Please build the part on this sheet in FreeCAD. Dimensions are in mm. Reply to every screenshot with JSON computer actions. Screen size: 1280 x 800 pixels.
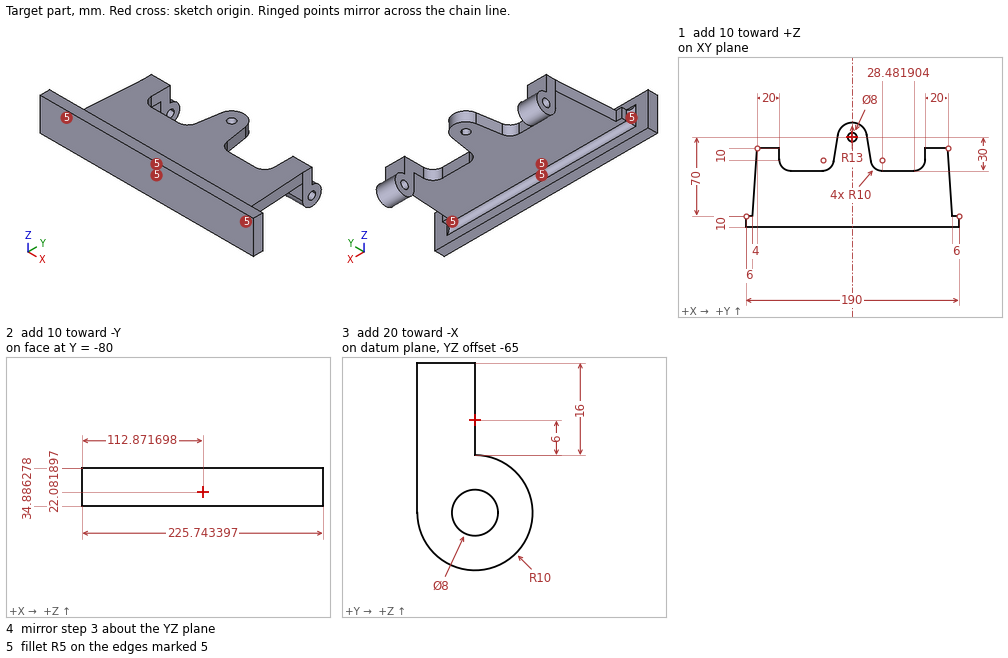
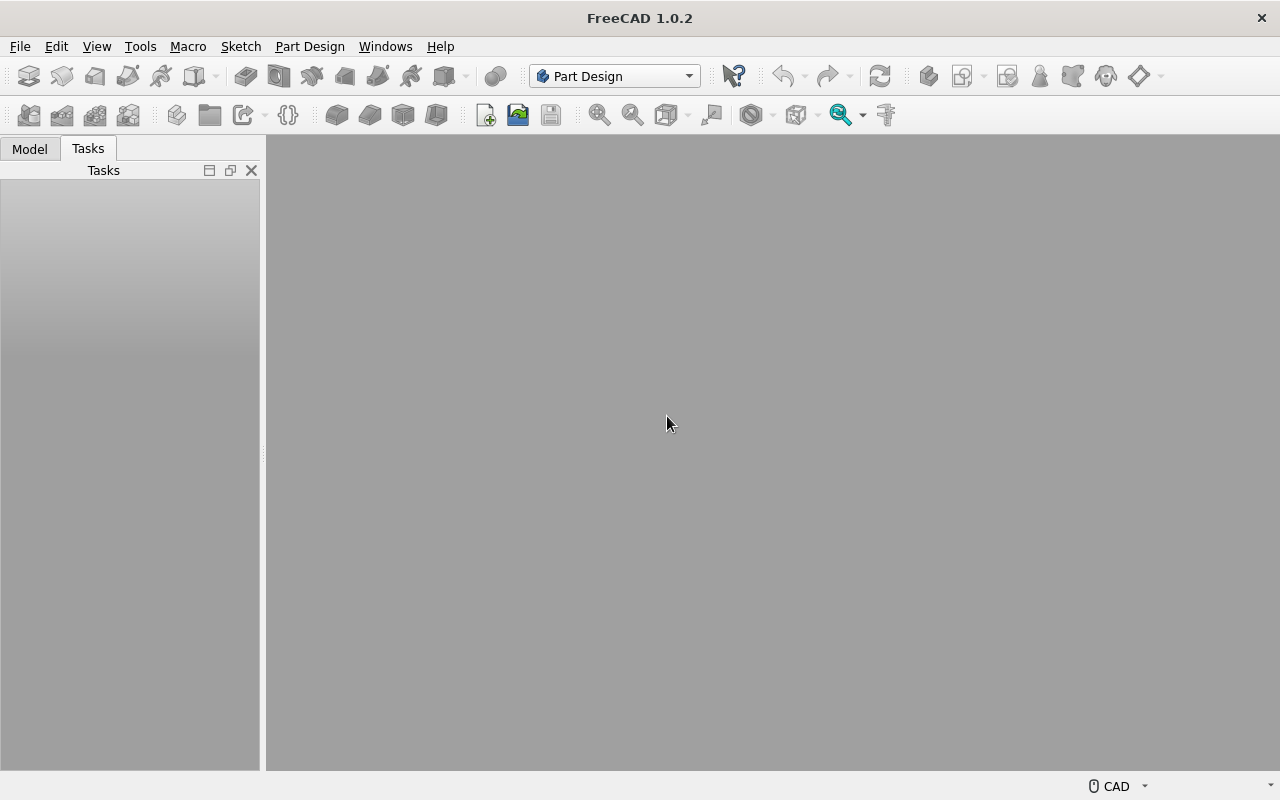
{"action": "left_click", "coordinate": [485, 116]}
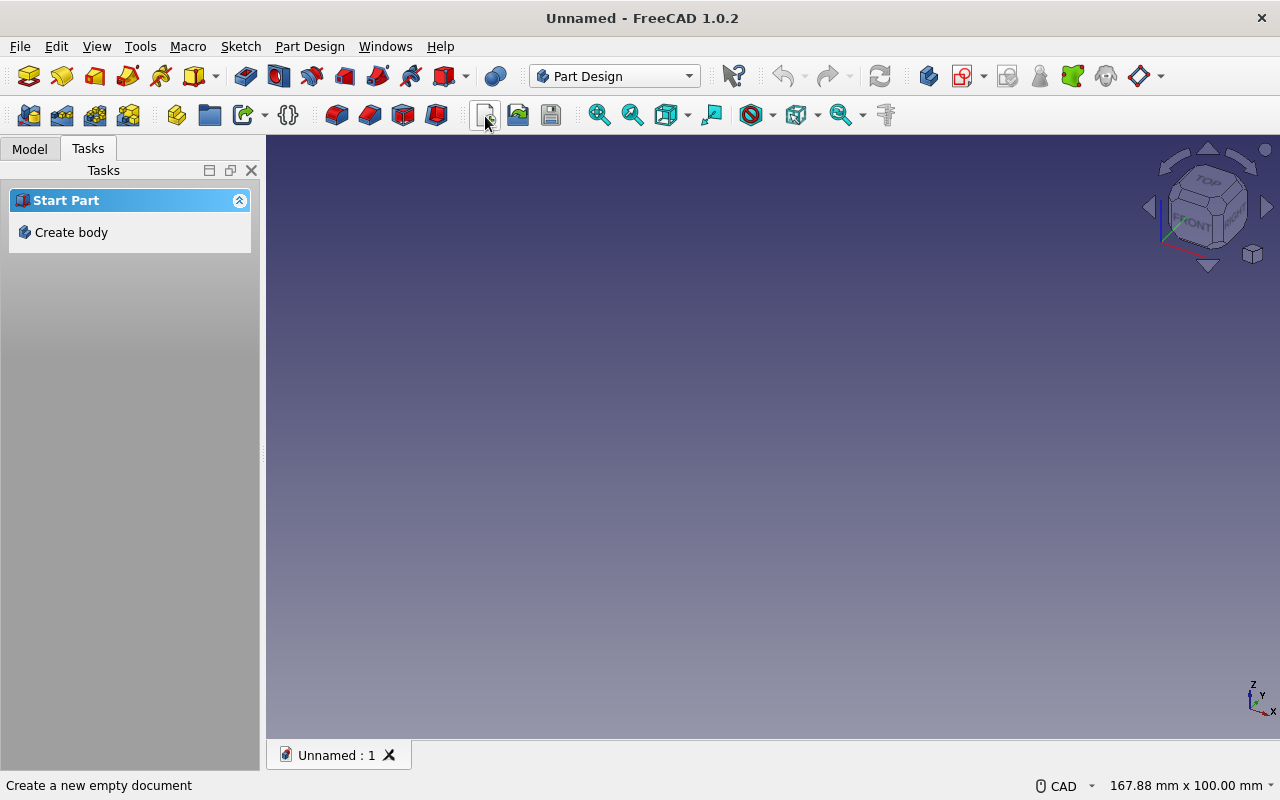
{"action": "left_click", "coordinate": [962, 76]}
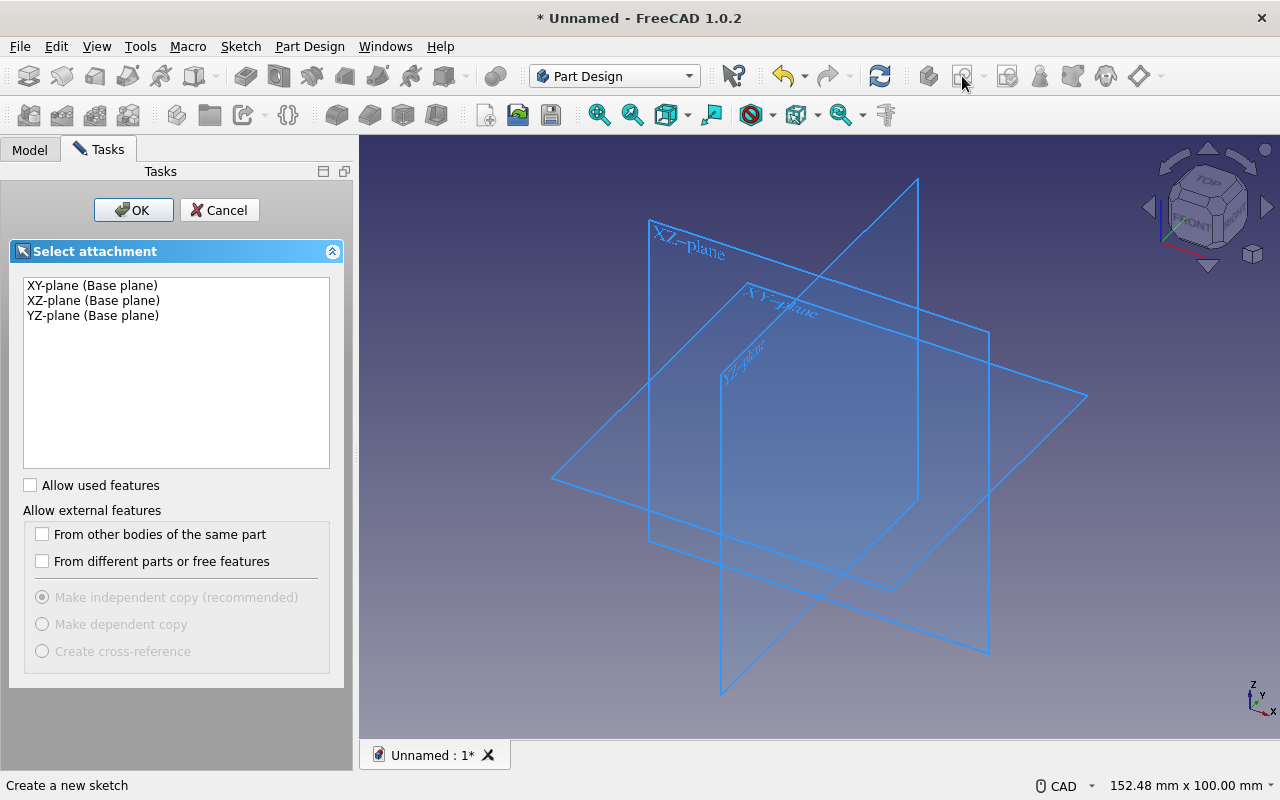
{"action": "left_click", "coordinate": [84, 286]}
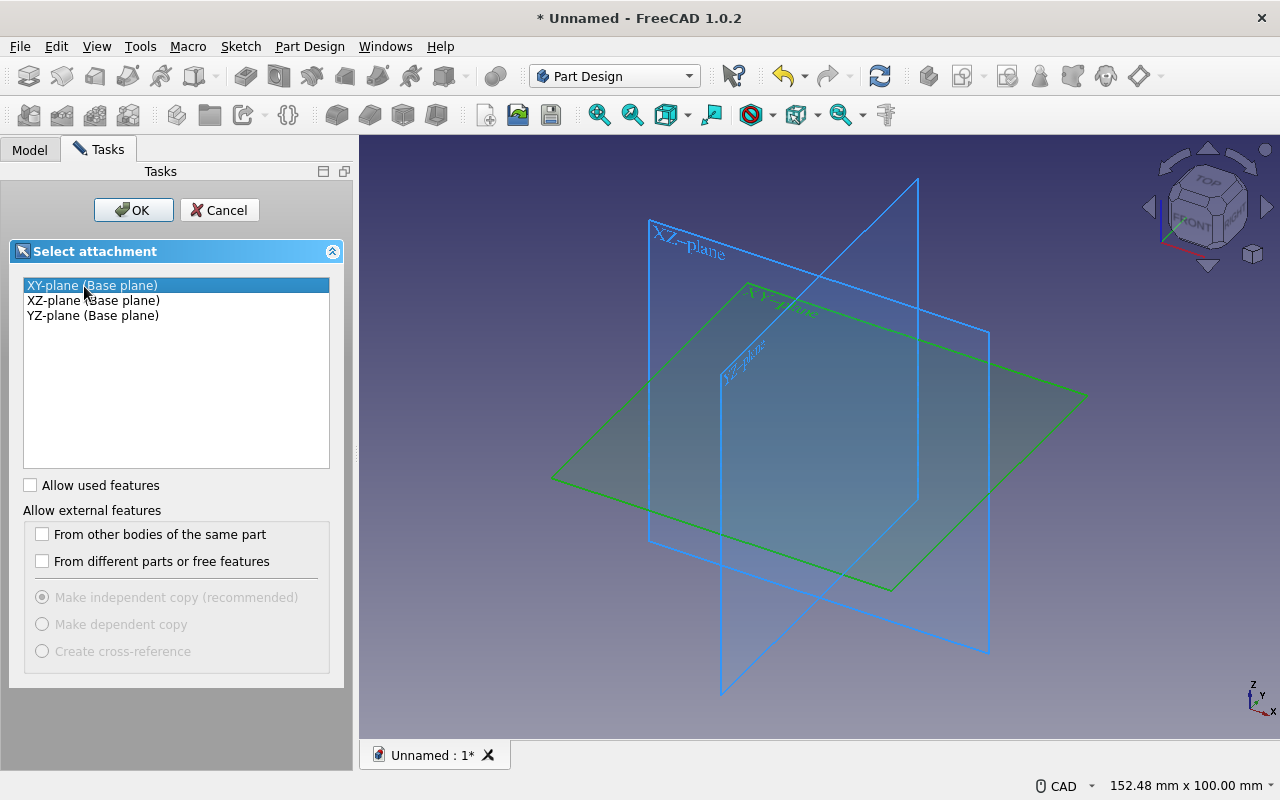
{"action": "left_click", "coordinate": [134, 210]}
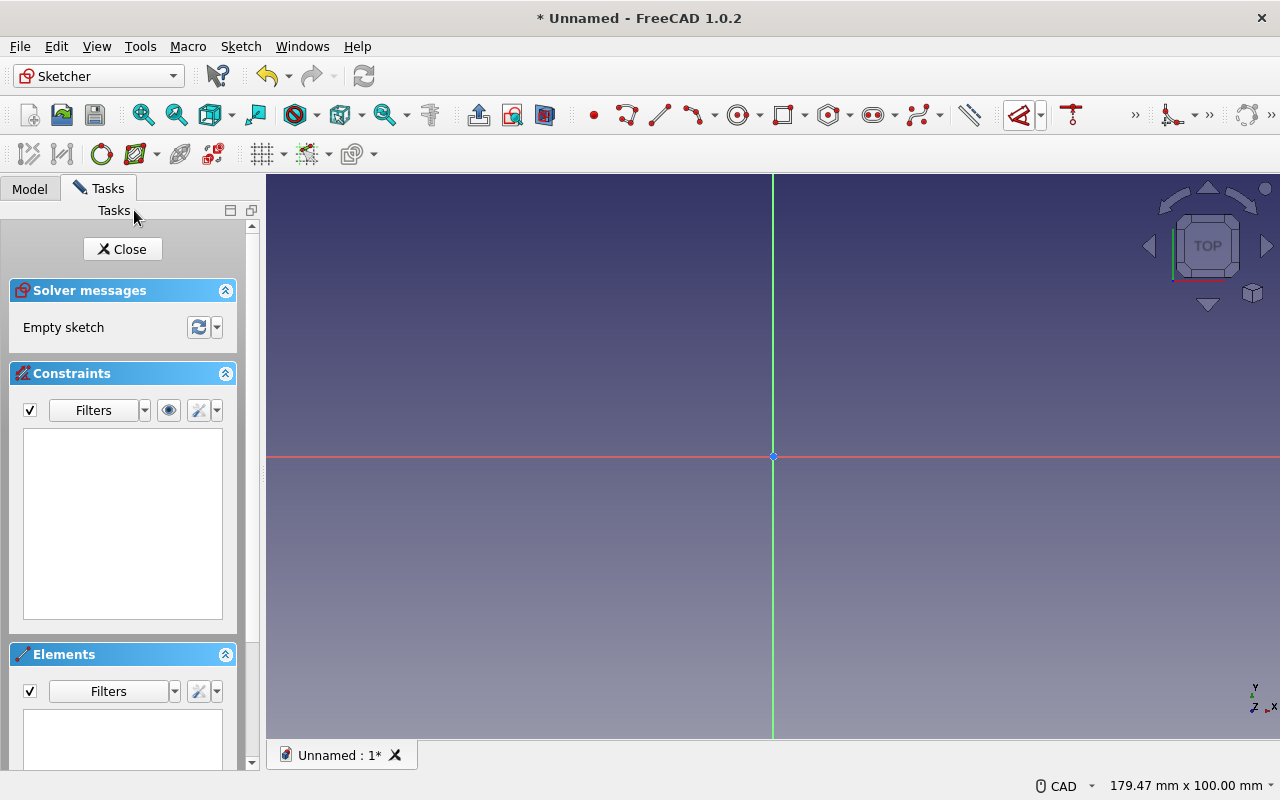
{"action": "scroll", "coordinate": [621, 226], "scroll_direction": "down", "scroll_amount": 3}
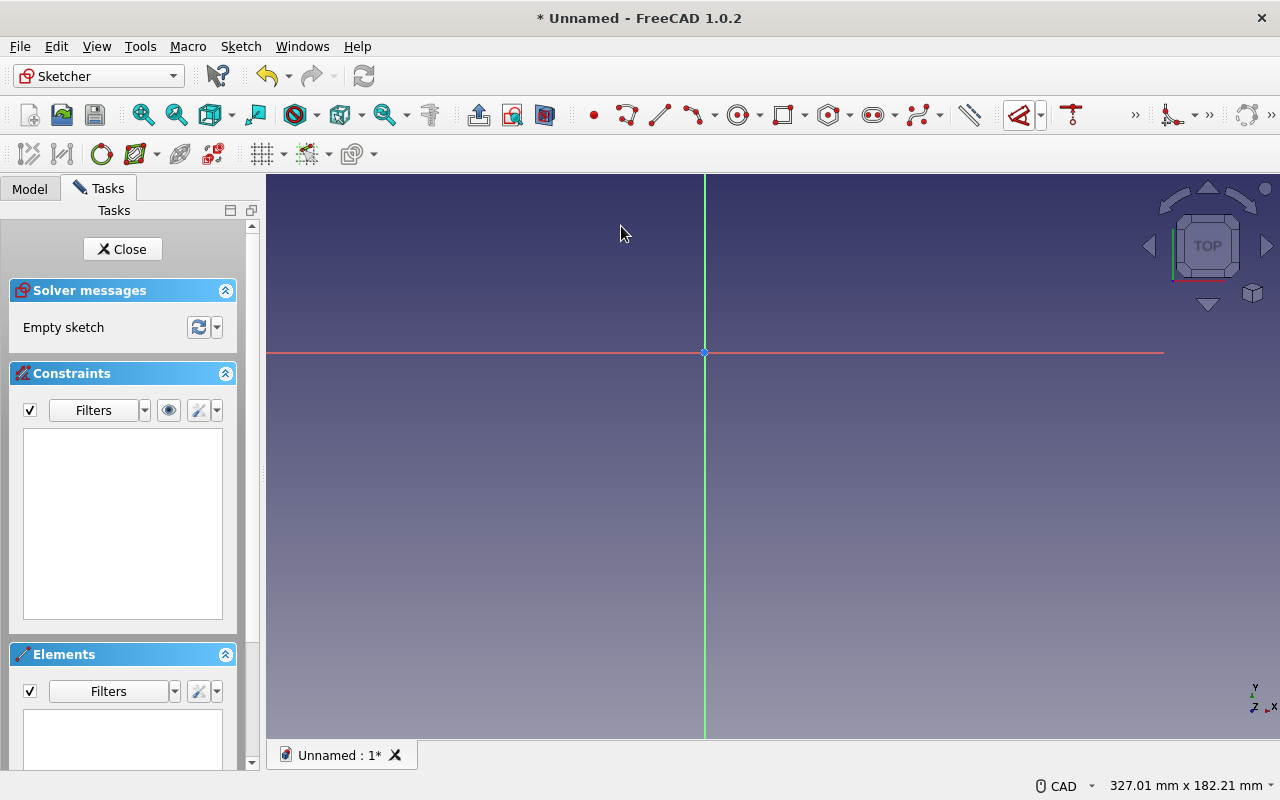
{"action": "left_click", "coordinate": [660, 116]}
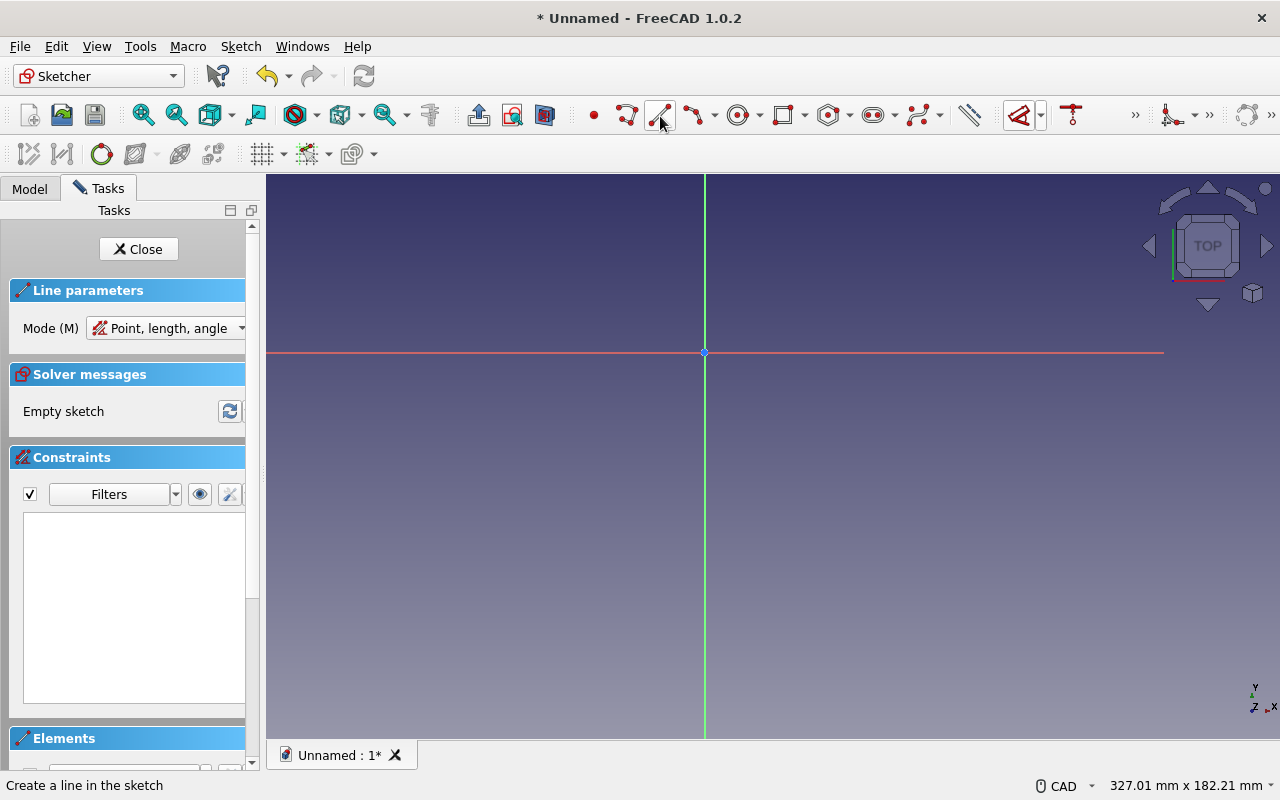
{"action": "left_click", "coordinate": [875, 446]}
{"action": "left_click", "coordinate": [787, 446]}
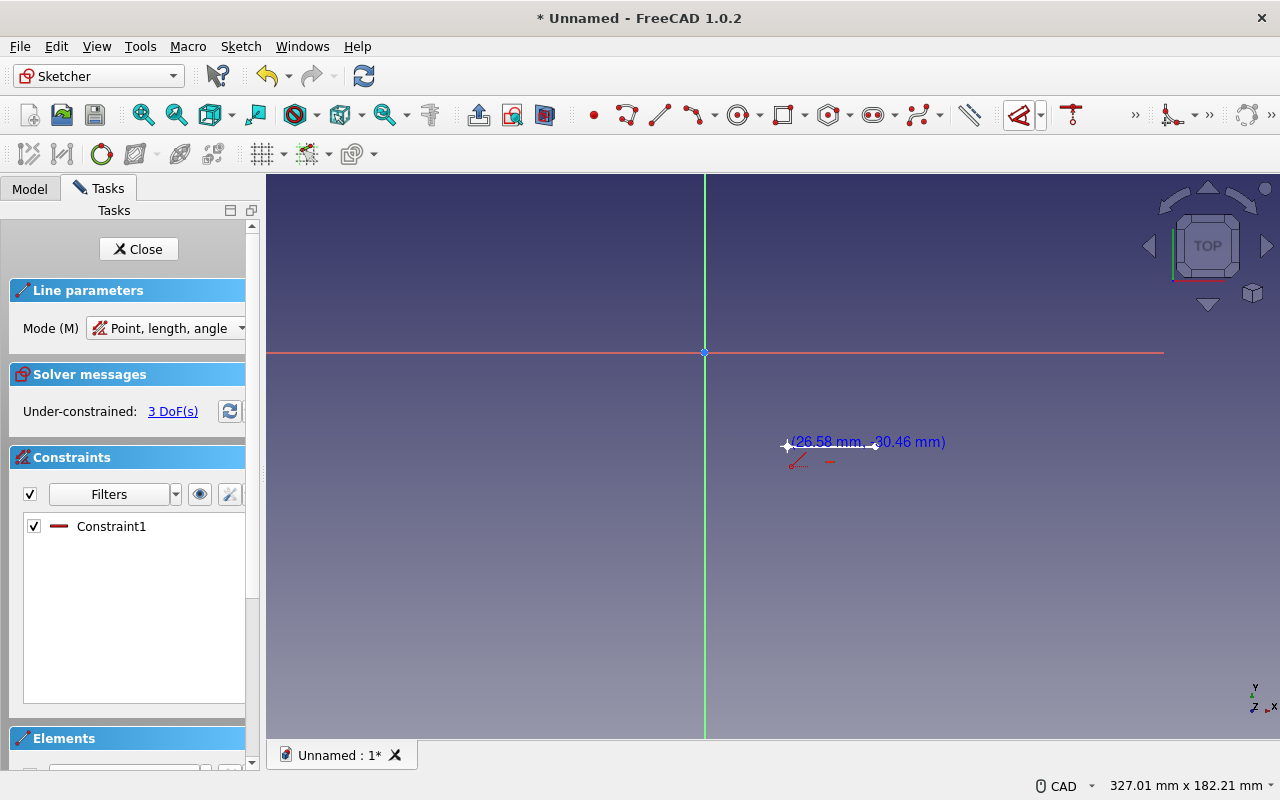
{"action": "left_click", "coordinate": [756, 419]}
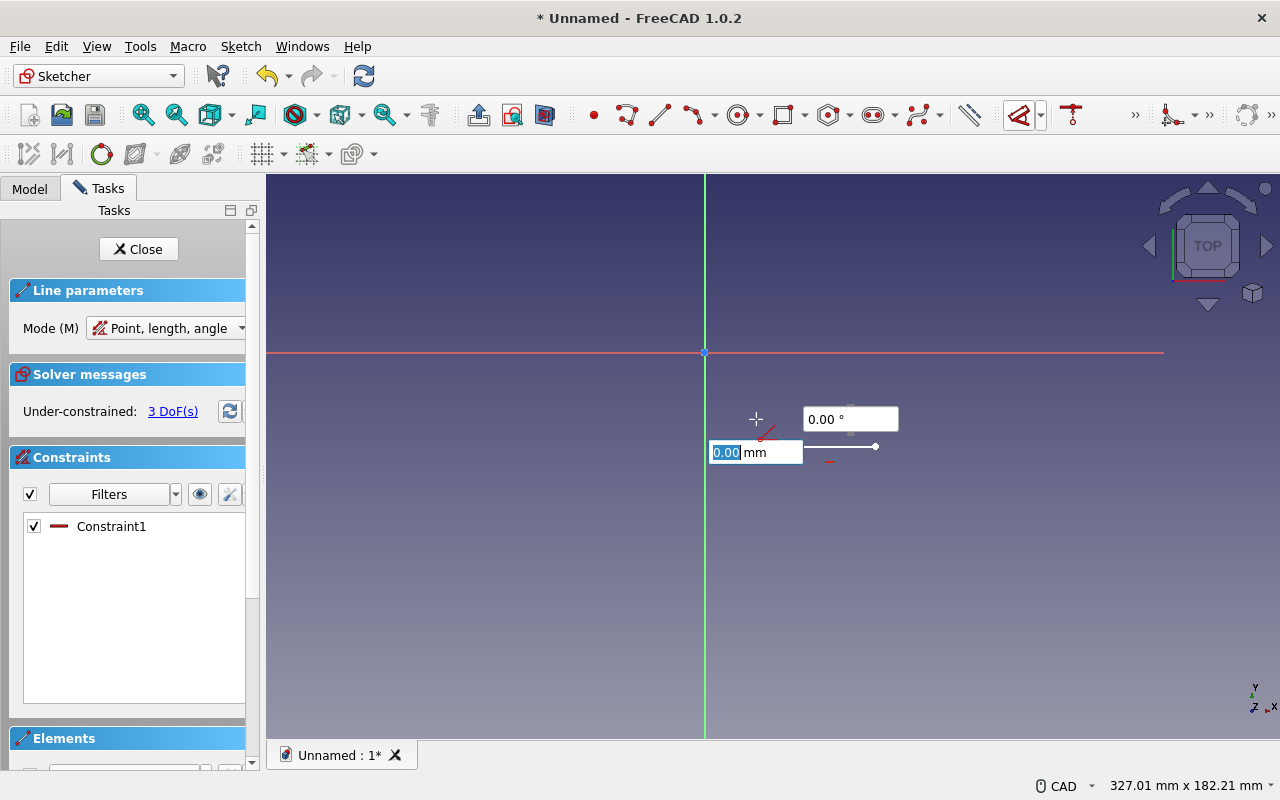
{"action": "scroll", "coordinate": [744, 346], "scroll_direction": "up", "scroll_amount": 5}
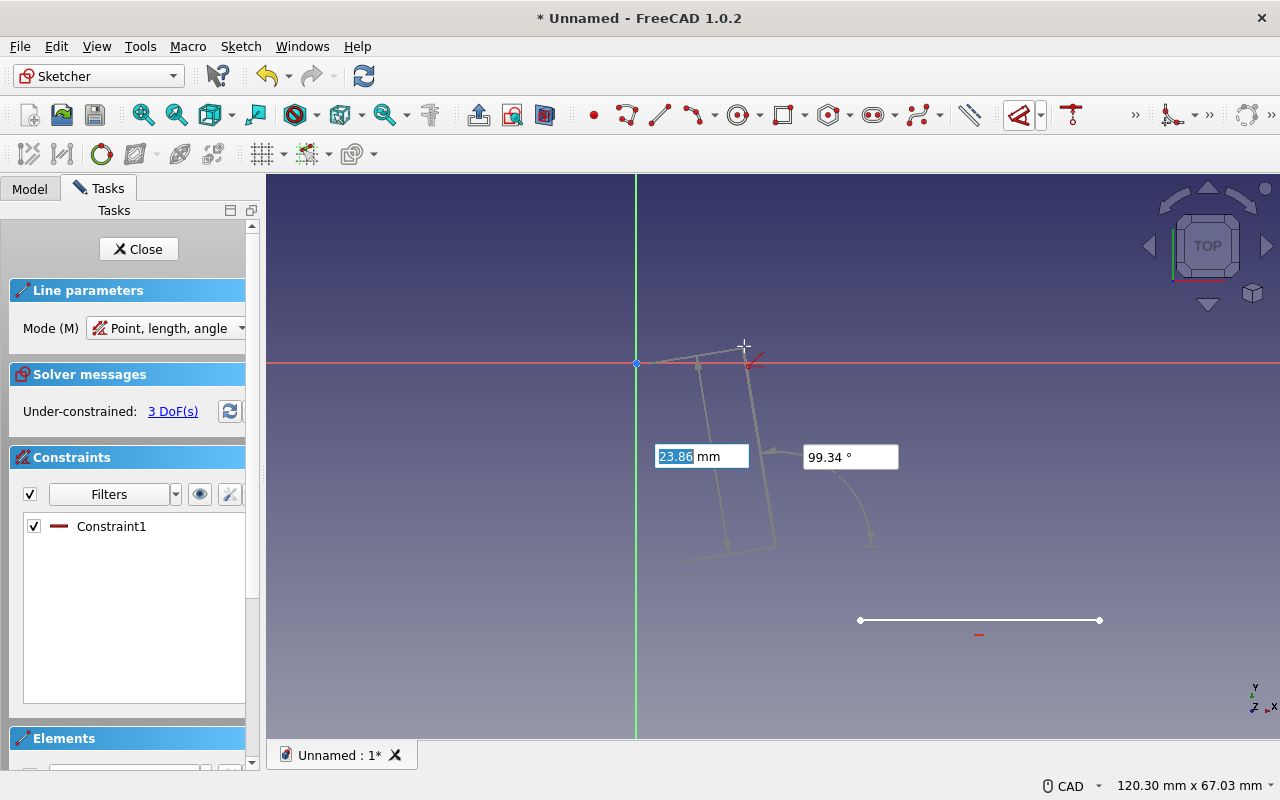
{"action": "left_click", "coordinate": [744, 346]}